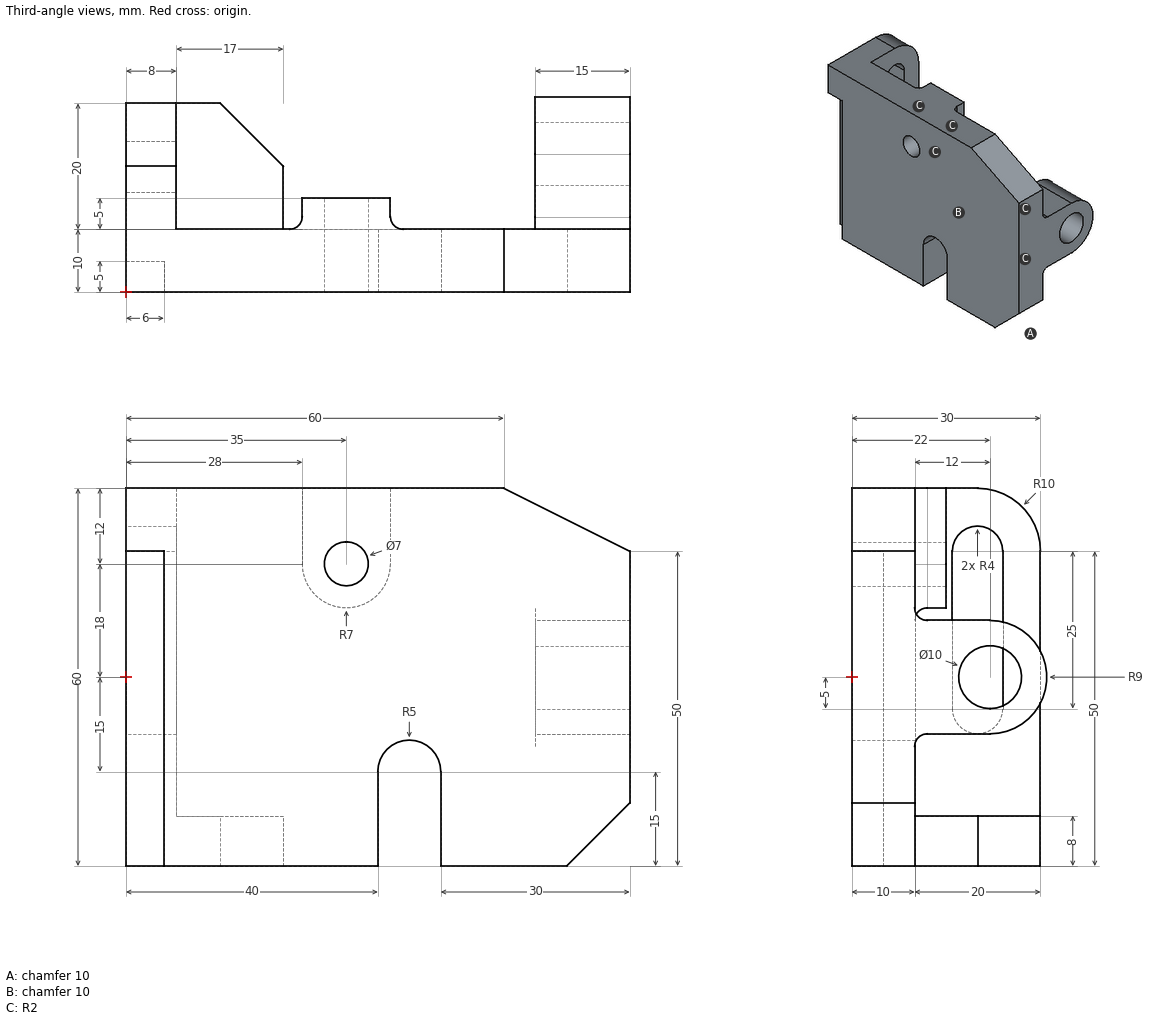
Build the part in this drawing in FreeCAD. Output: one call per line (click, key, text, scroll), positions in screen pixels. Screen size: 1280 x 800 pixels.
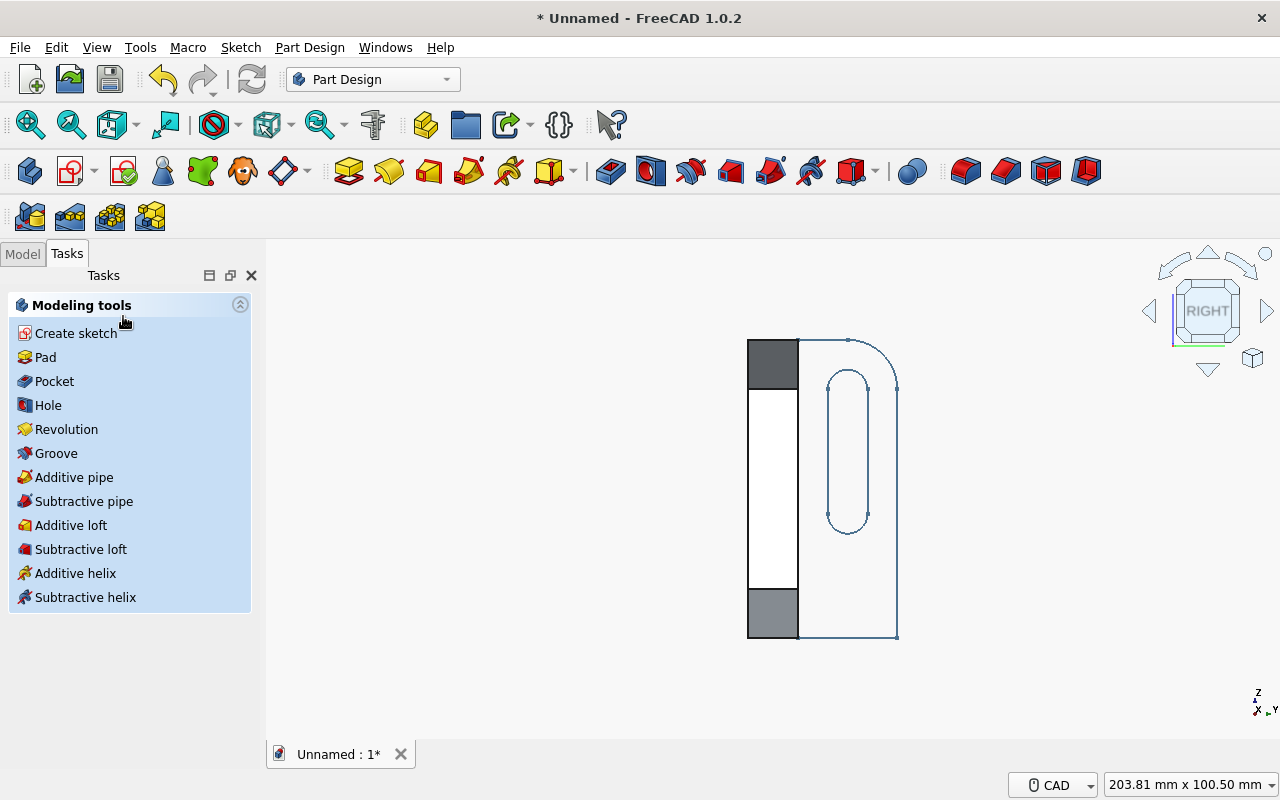
click(350, 172)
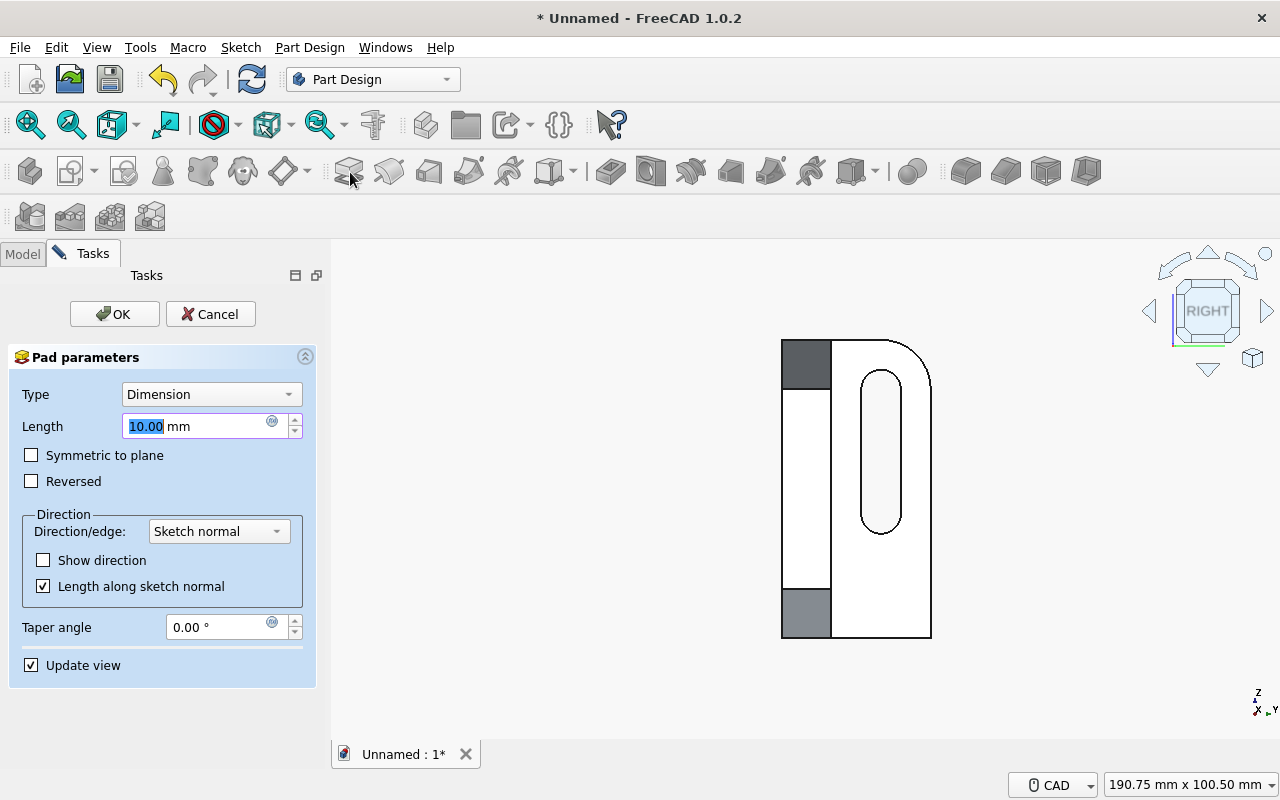
text(8)
key(Tab)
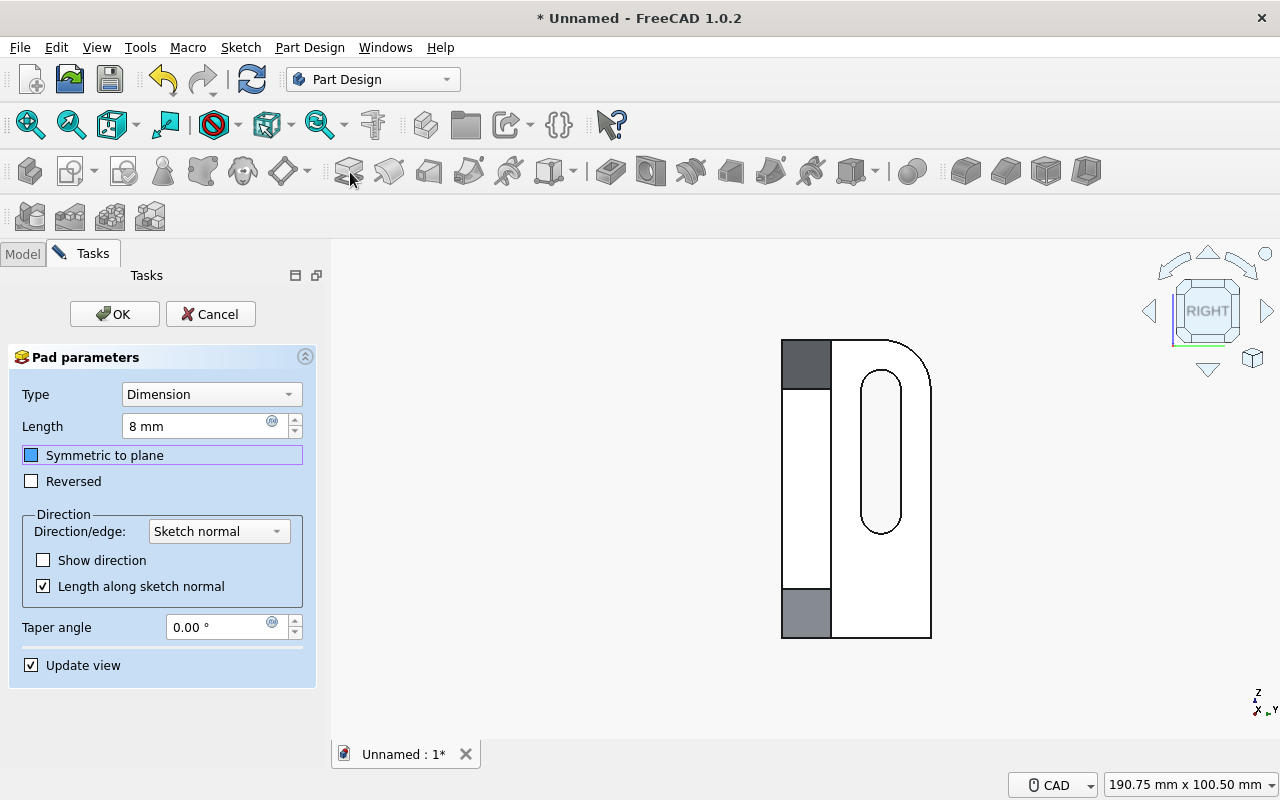
click(115, 314)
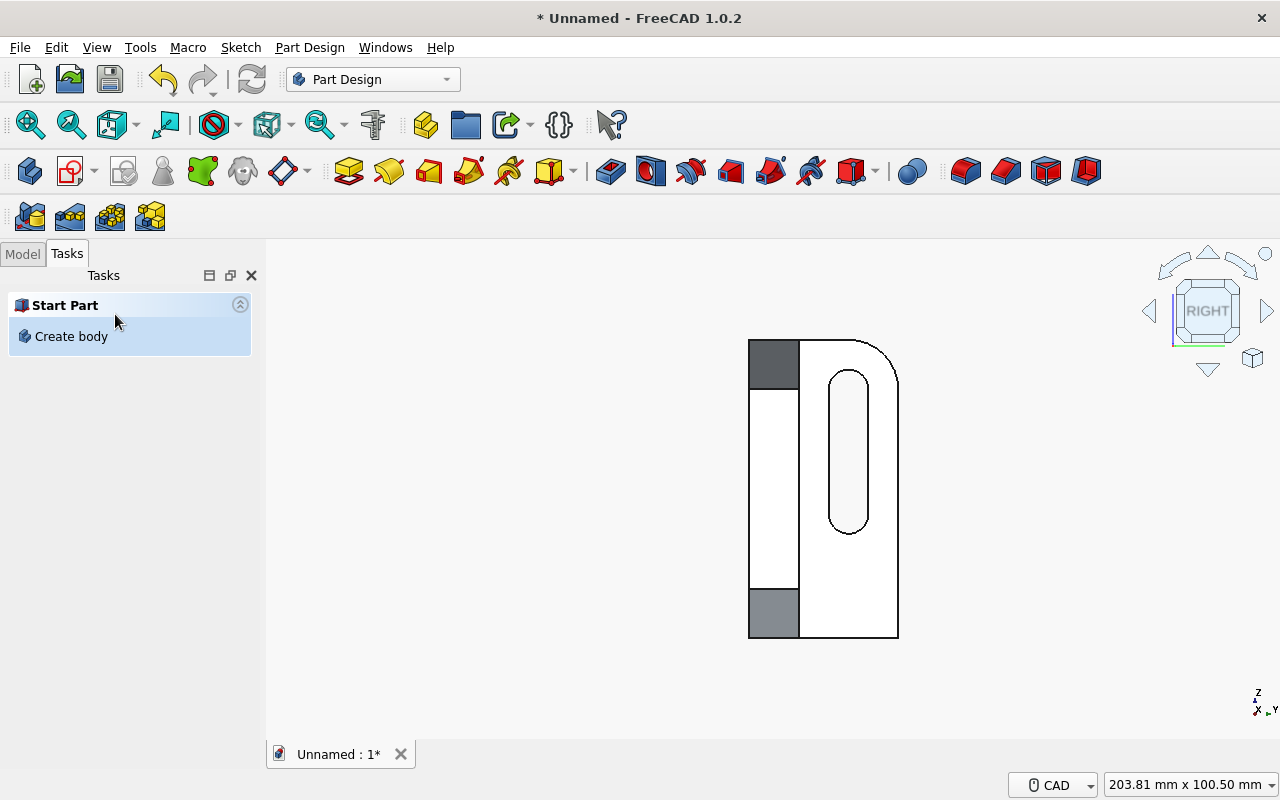
key(5)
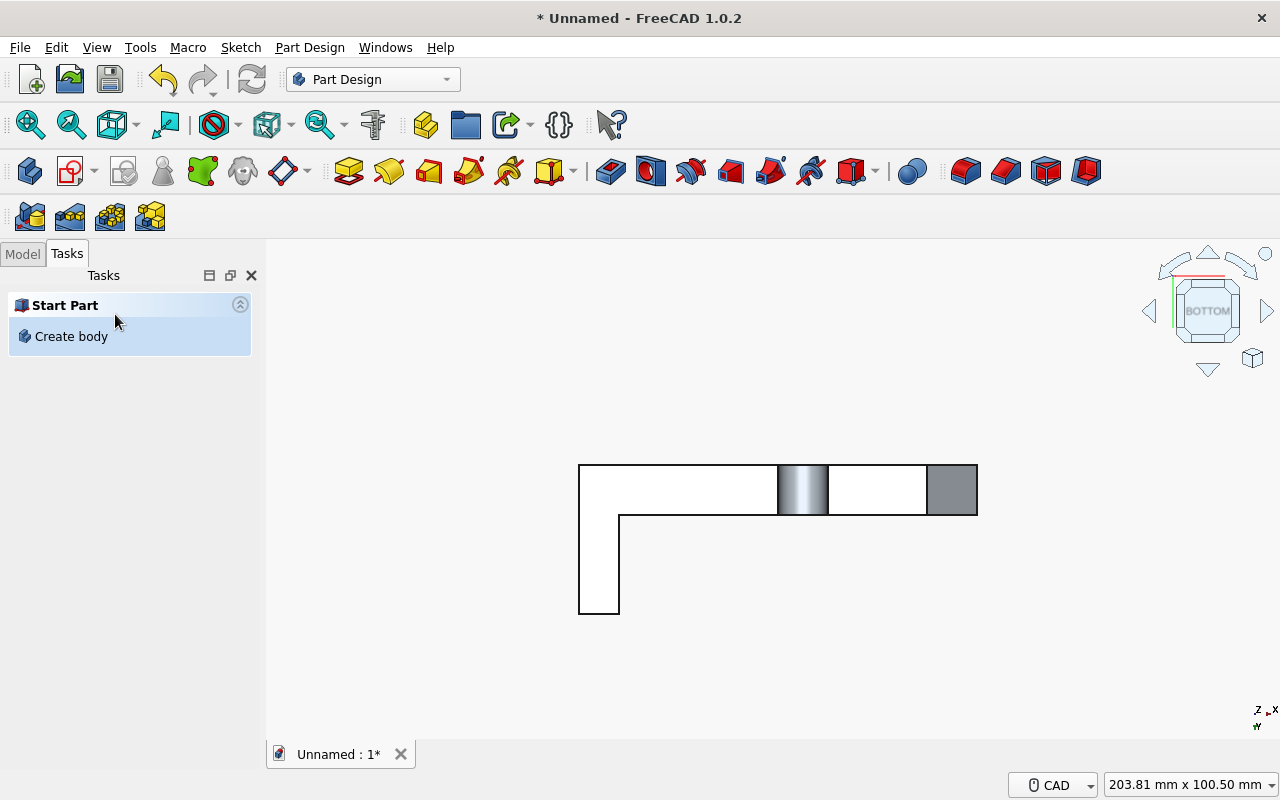
key(v)
key(f)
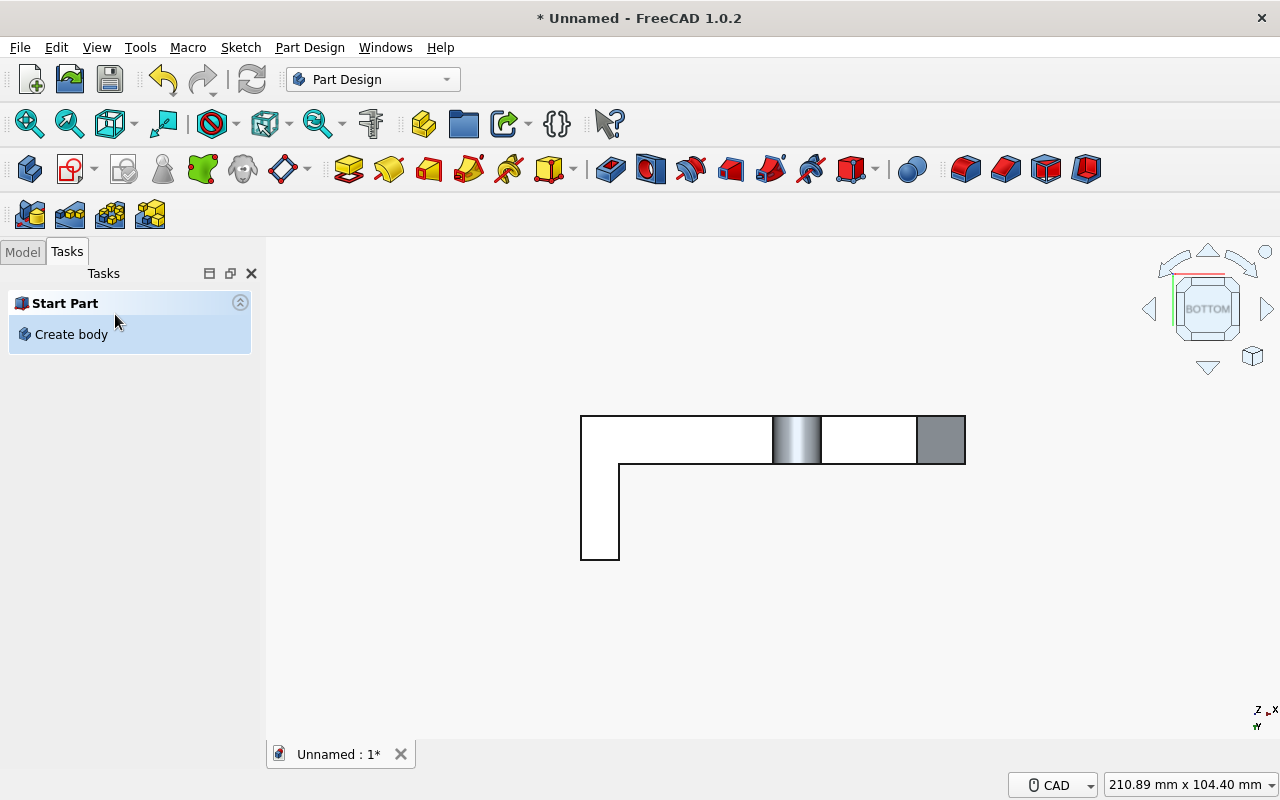
click(732, 446)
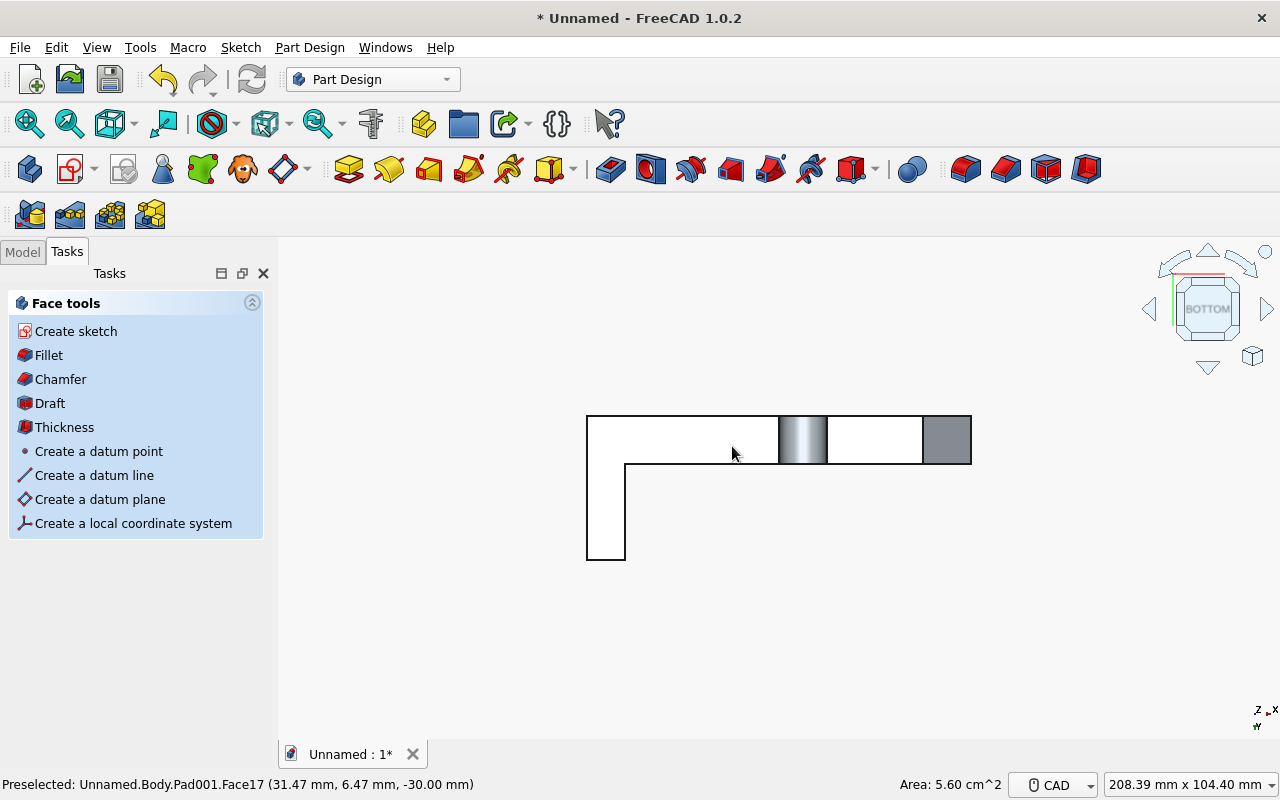
click(70, 170)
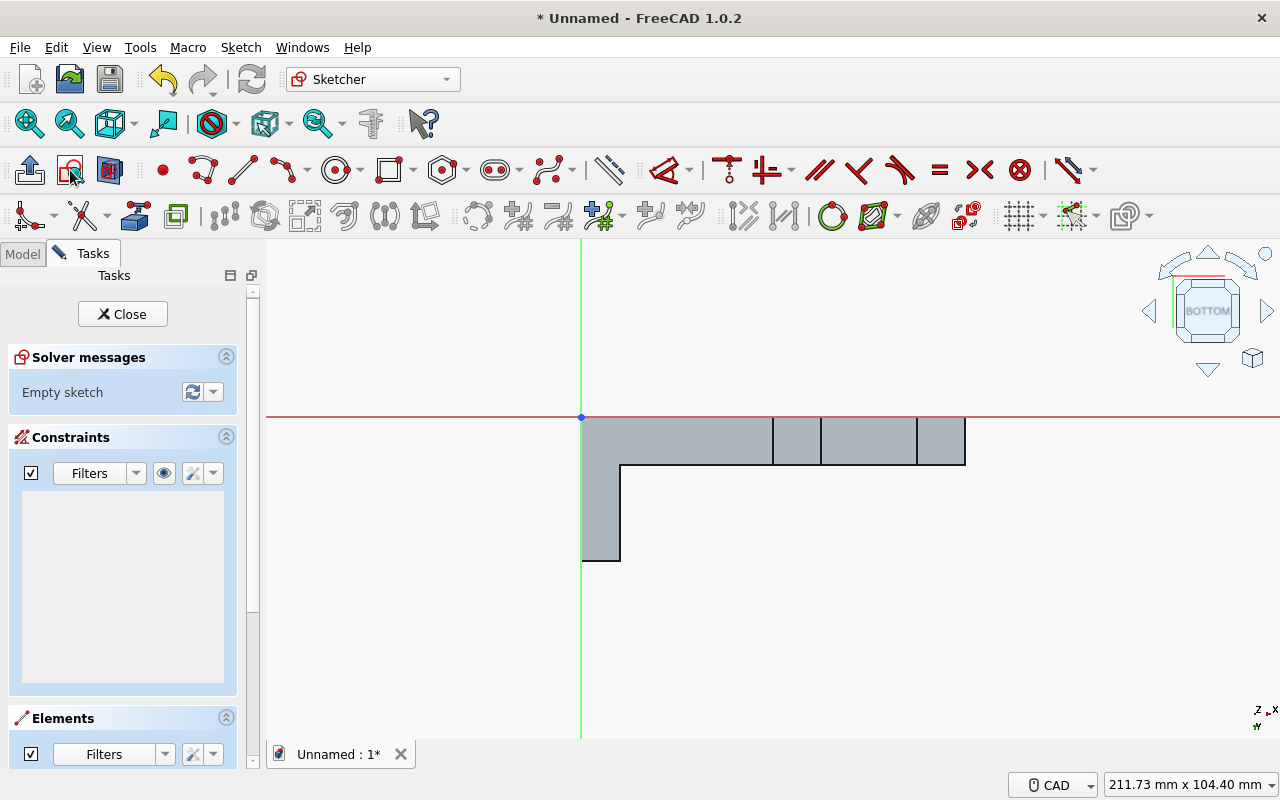
scroll(590, 489, up, 4)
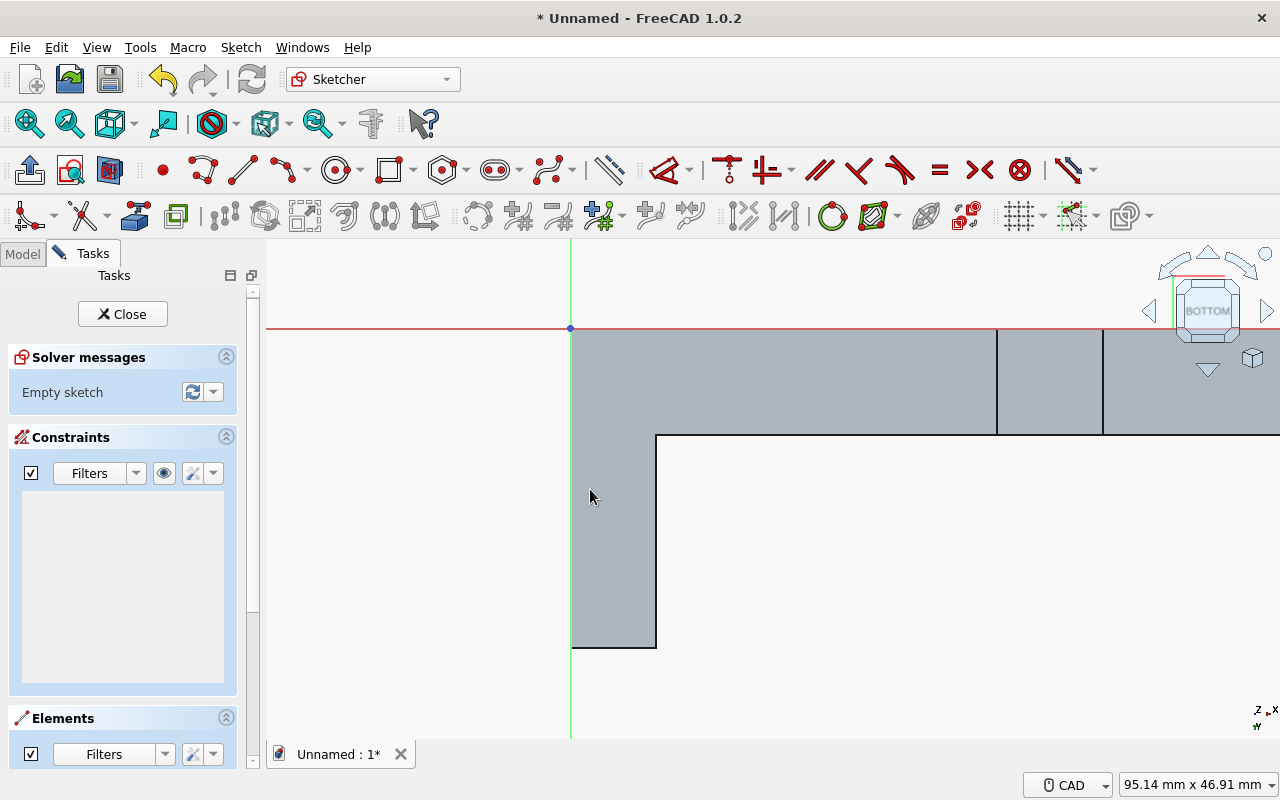
key(g)
key(r)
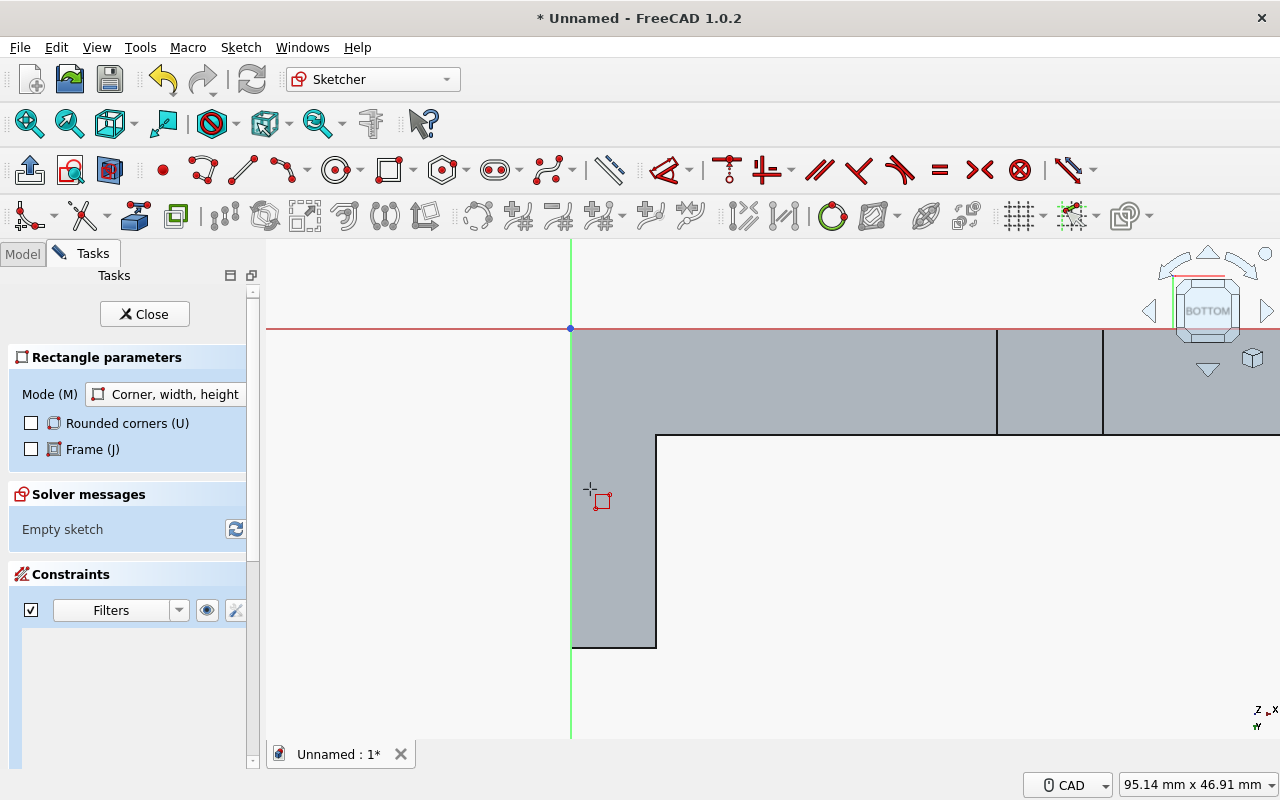
click(656, 435)
click(837, 648)
key(Escape)